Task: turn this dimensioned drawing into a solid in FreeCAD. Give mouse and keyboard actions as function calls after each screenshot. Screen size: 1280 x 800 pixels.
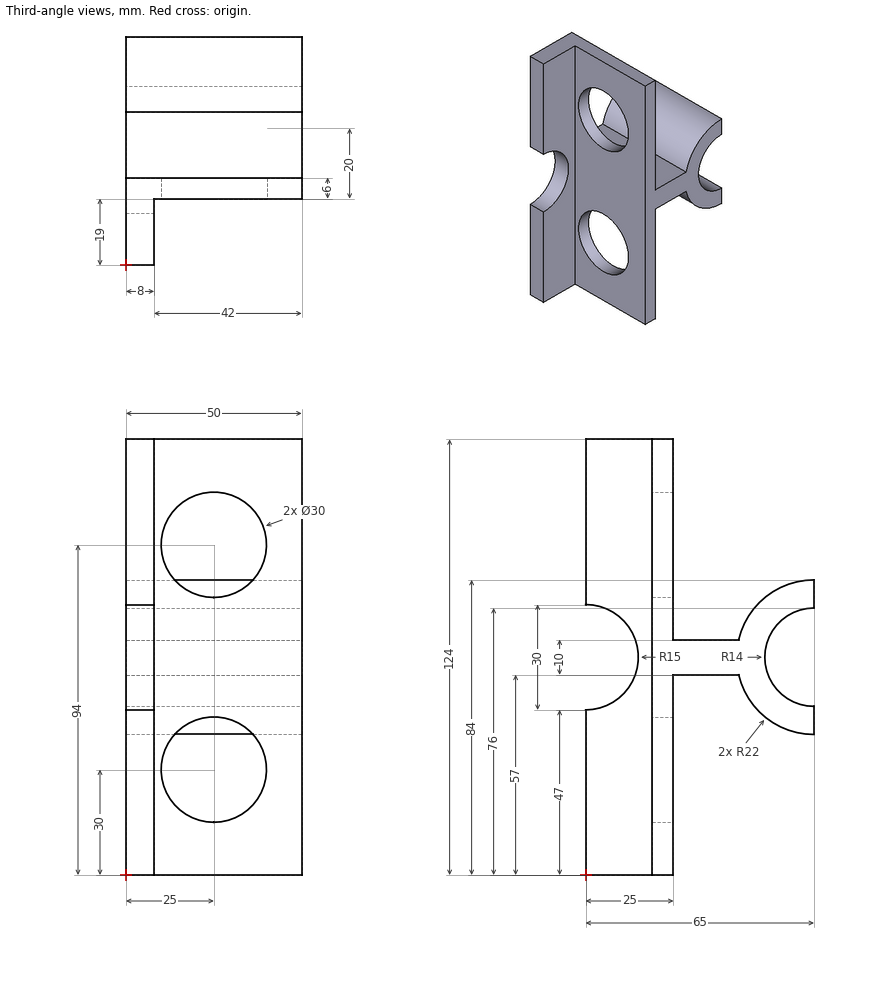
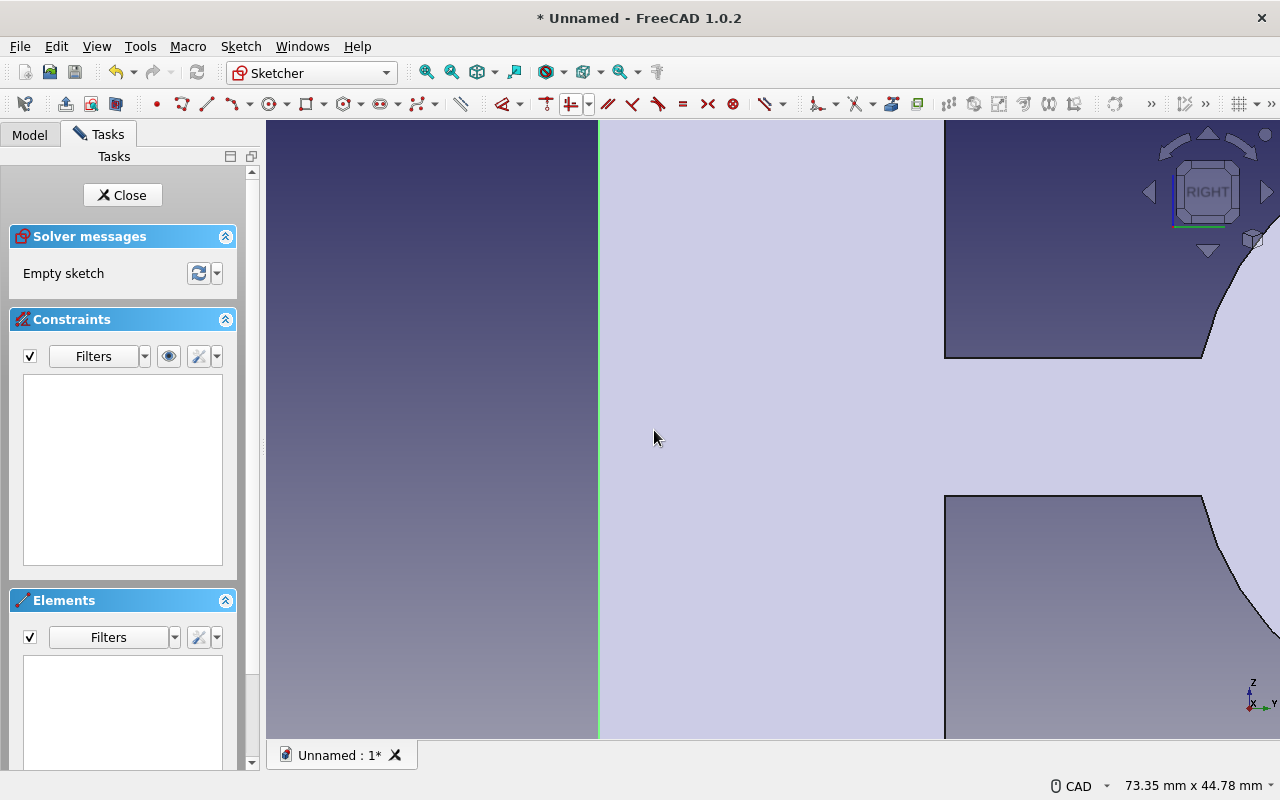
key(g)
key(l)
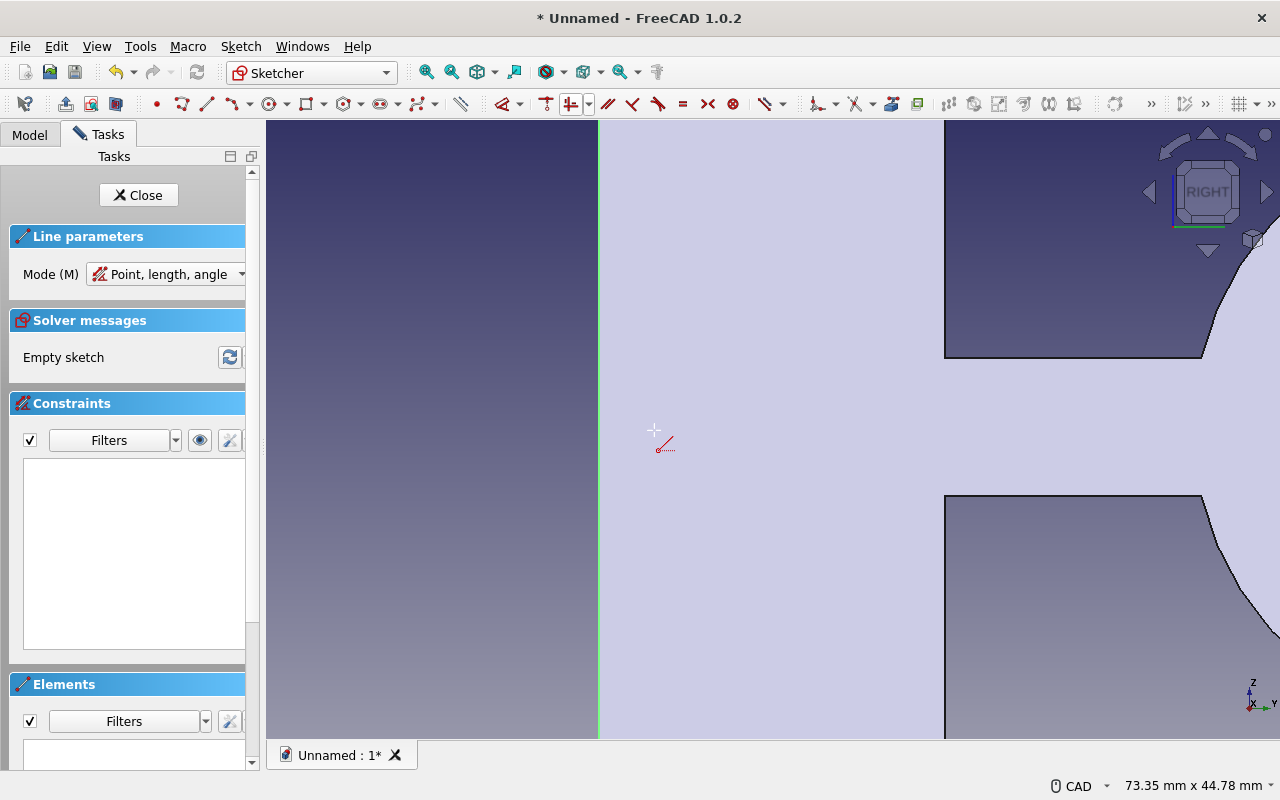
click(599, 635)
click(608, 220)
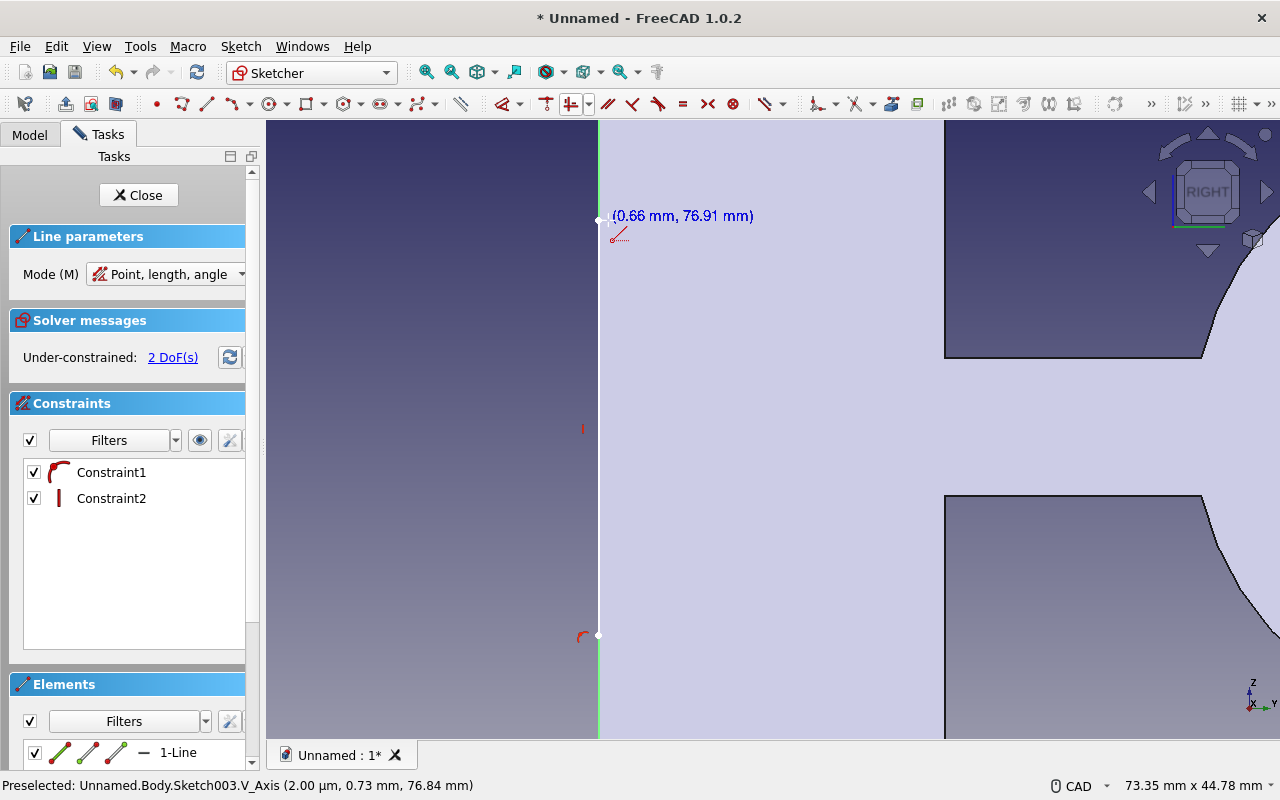
key(g)
key(3)
key(a)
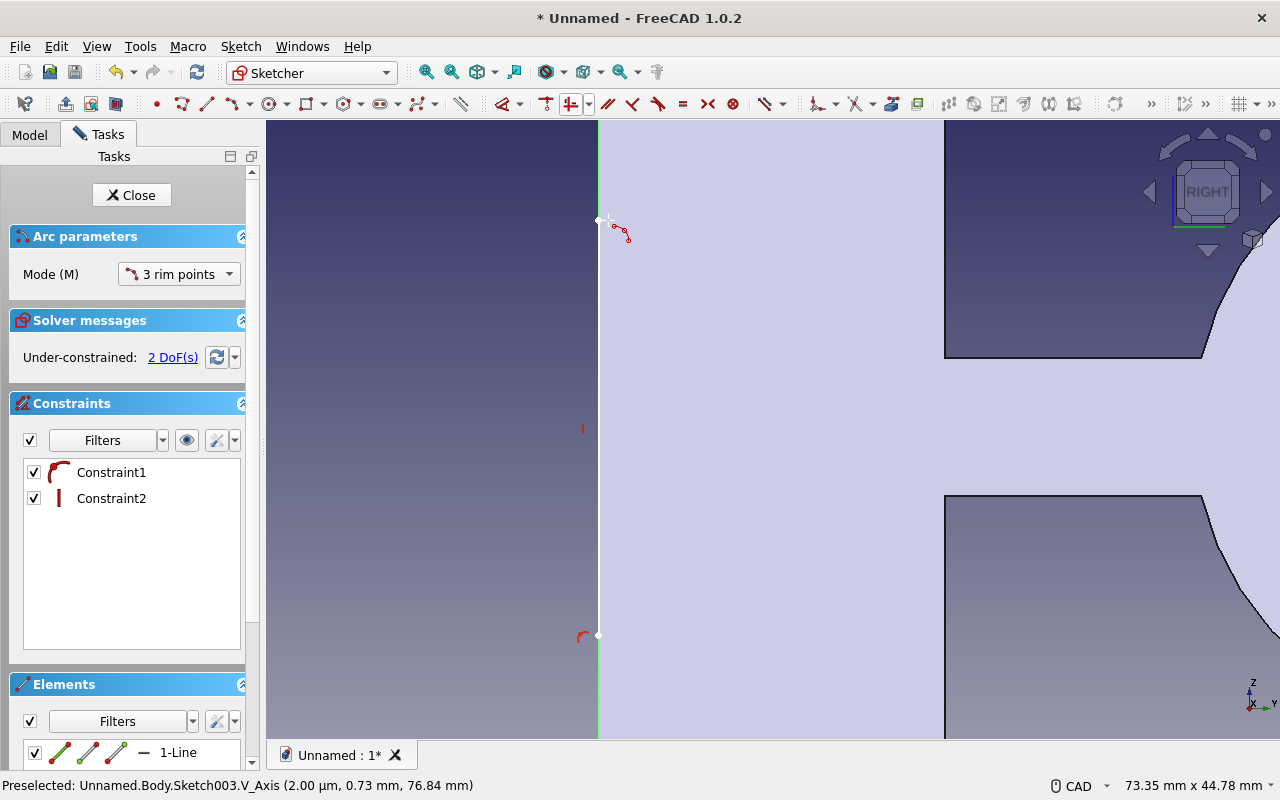
click(608, 220)
click(599, 636)
click(806, 427)
key(Escape)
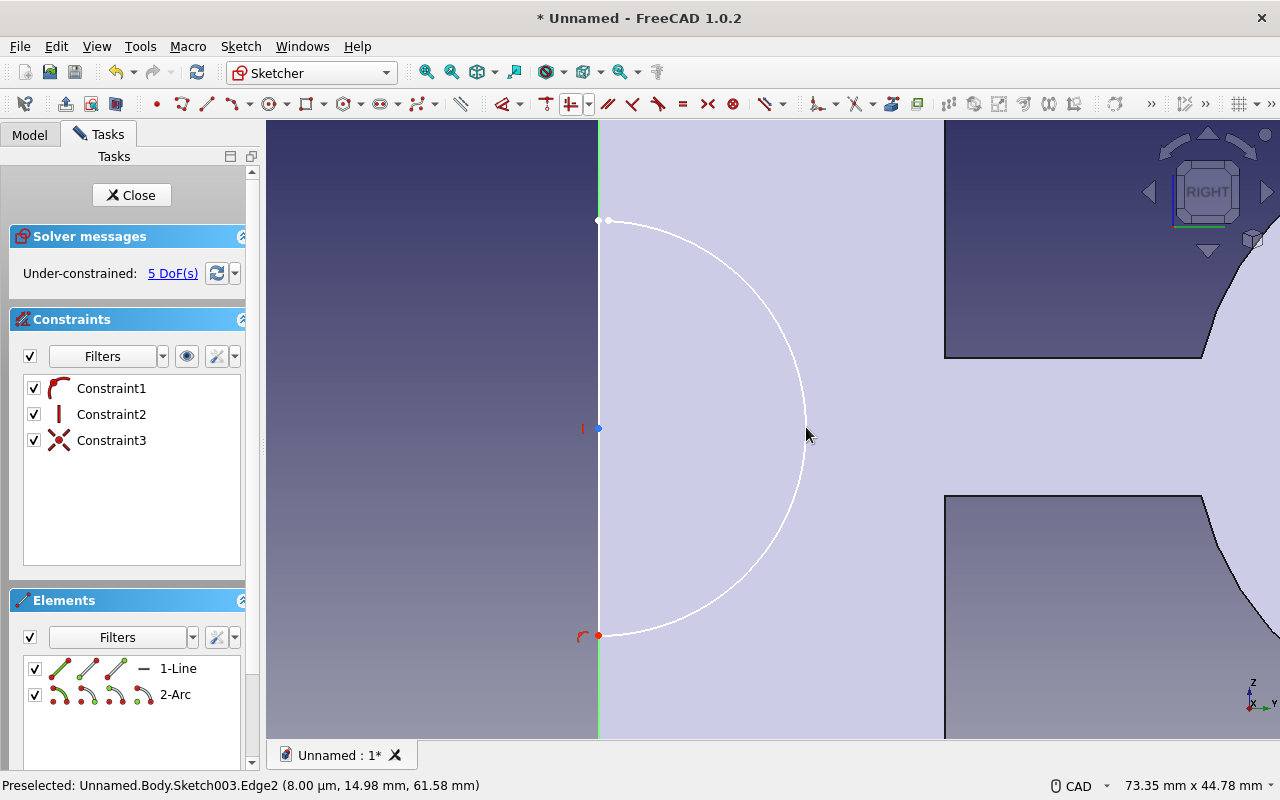
click(598, 428)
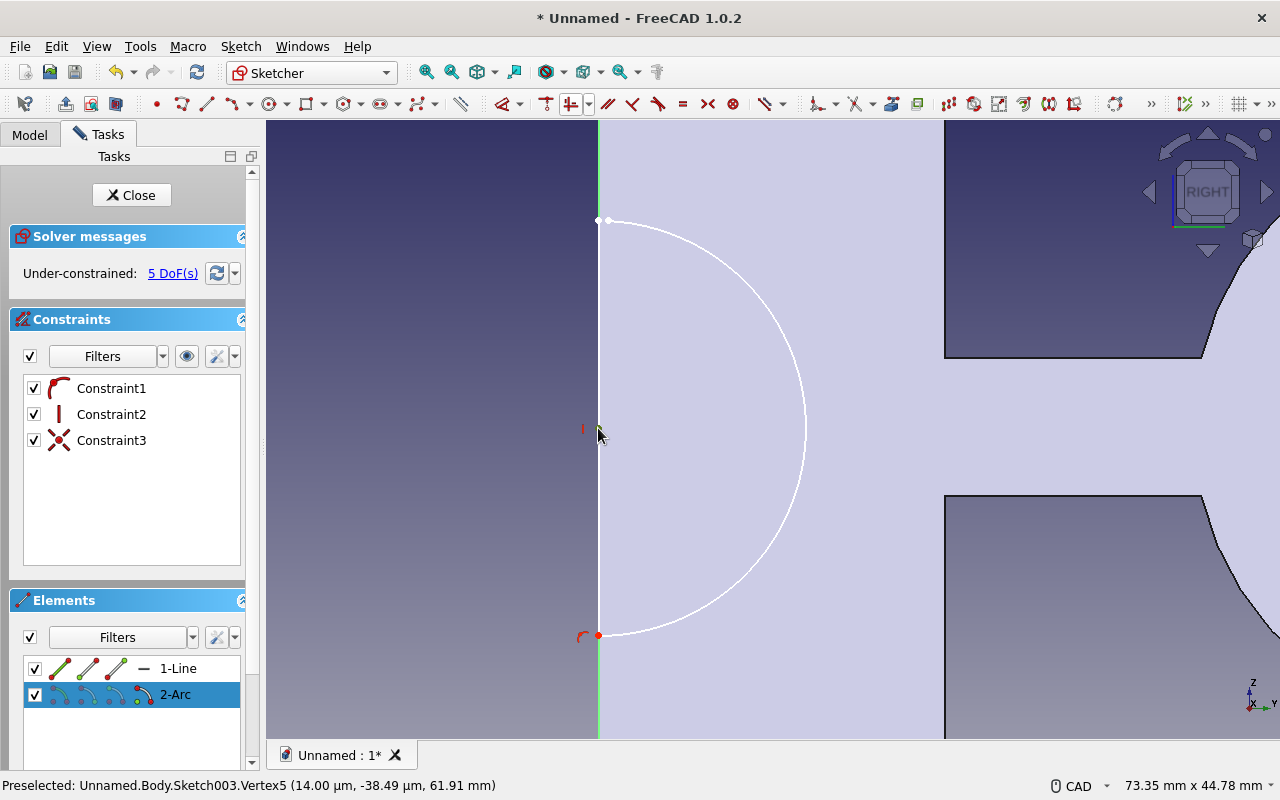
click(599, 671)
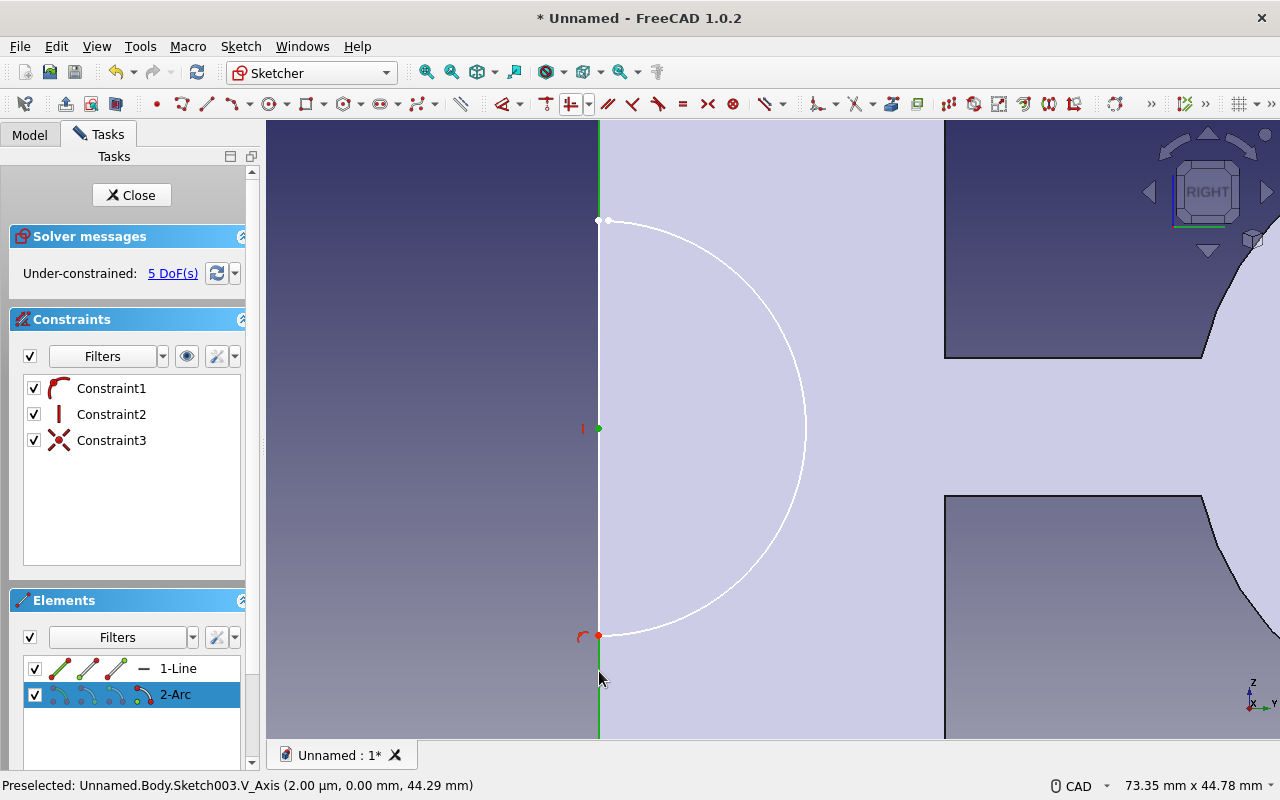
click(546, 104)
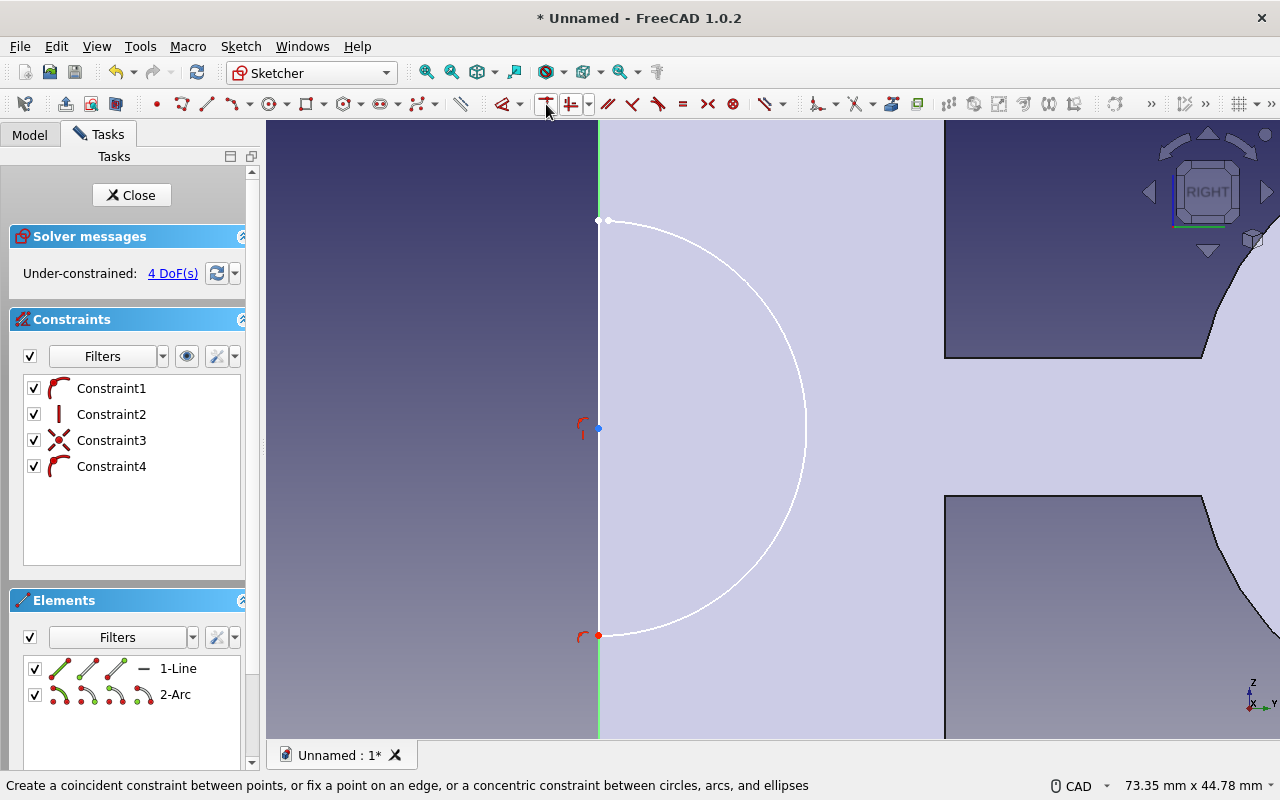
key(d)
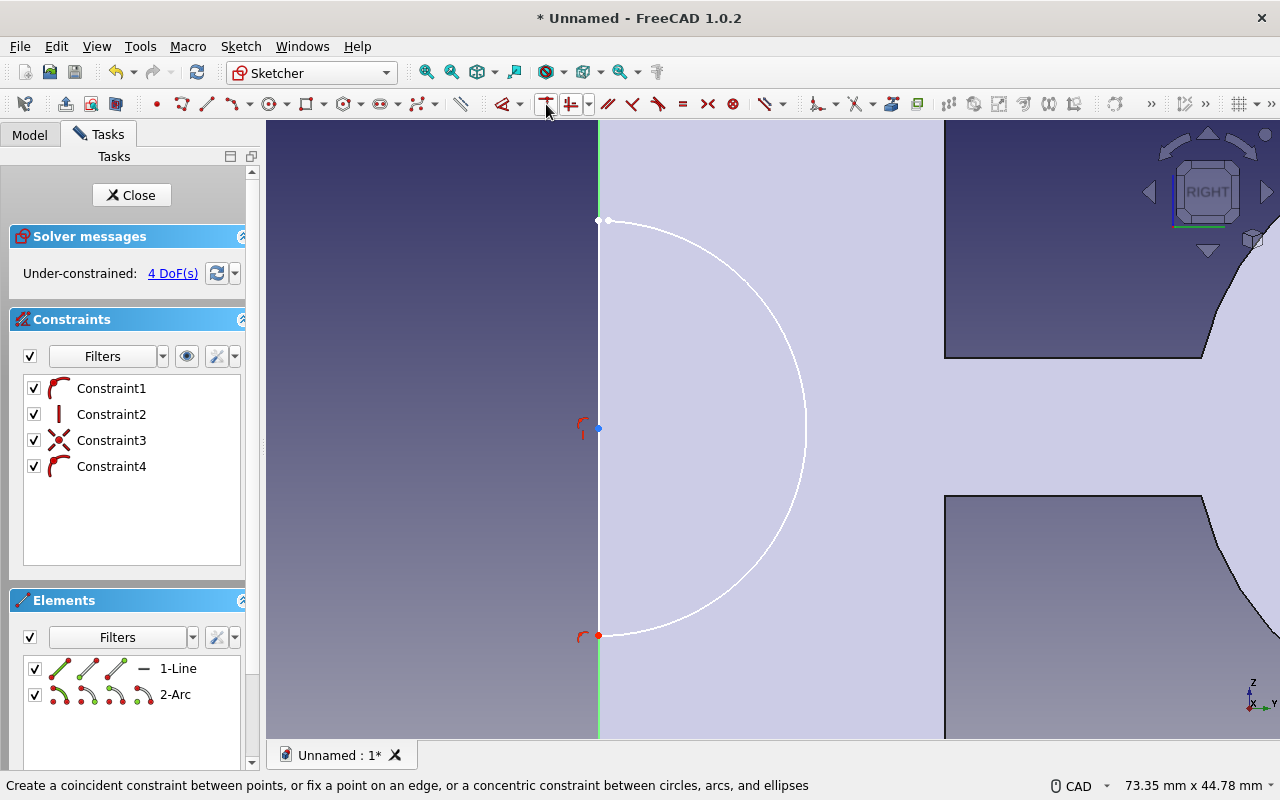
click(765, 553)
click(791, 572)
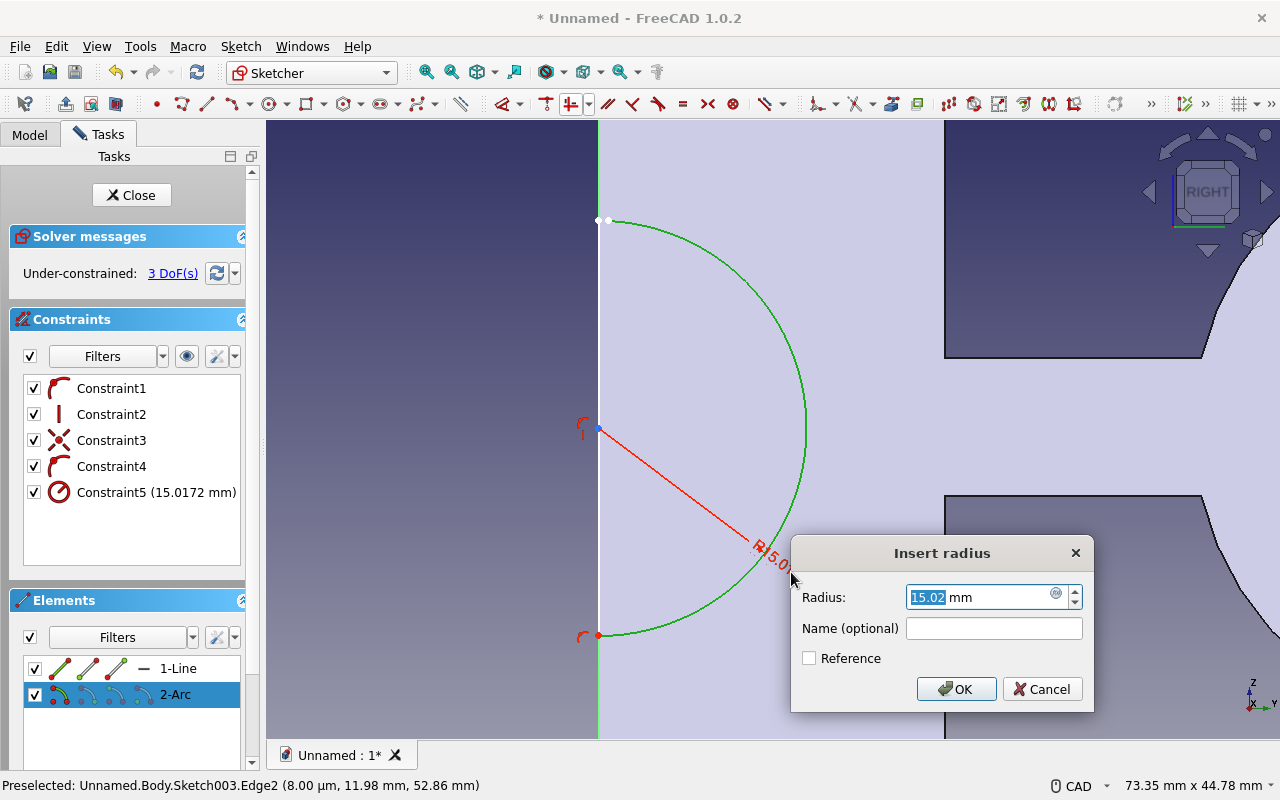
text(15)
key(Return)
key(Escape)